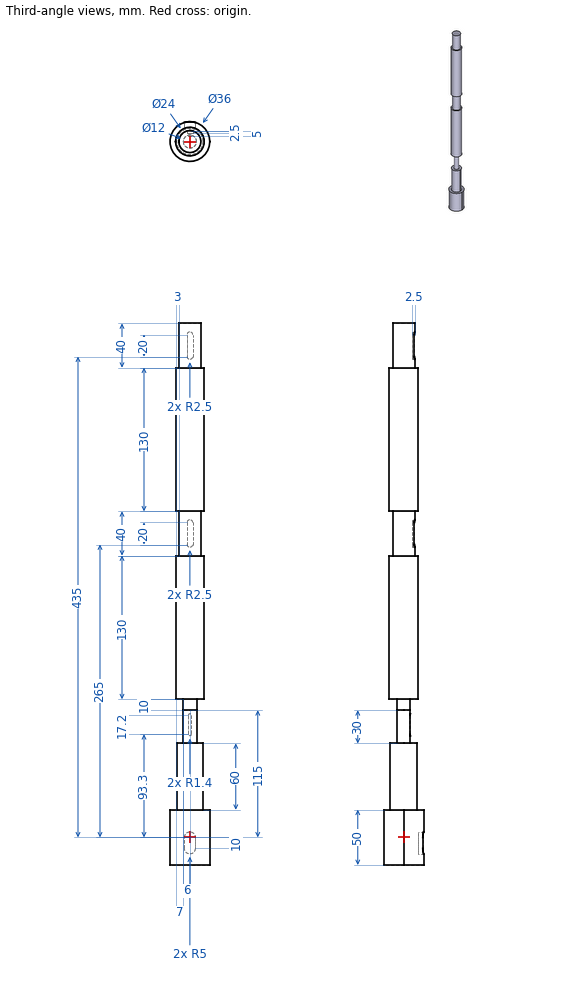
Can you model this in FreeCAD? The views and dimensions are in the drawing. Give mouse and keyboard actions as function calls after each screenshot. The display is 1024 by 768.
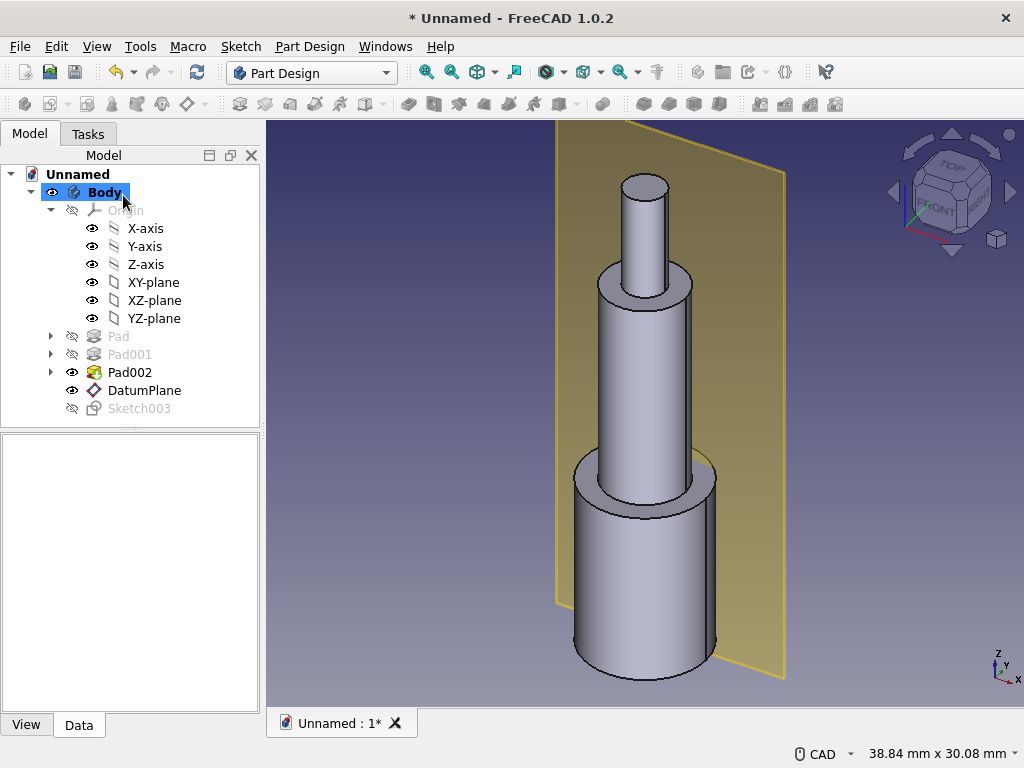
click(409, 104)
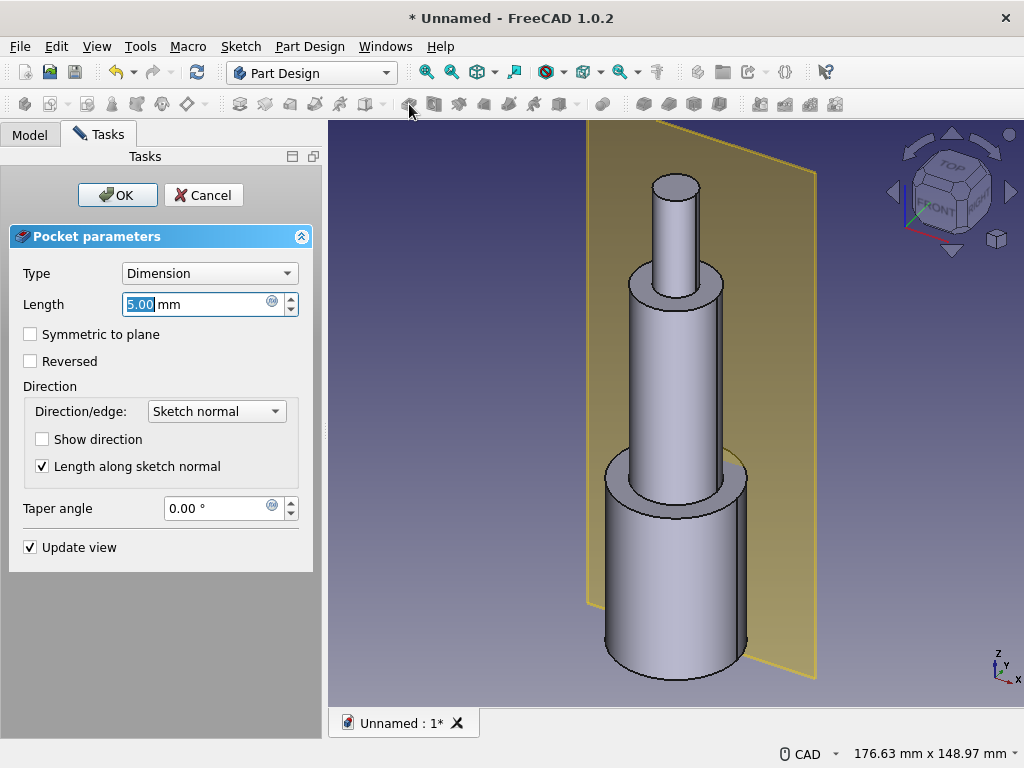
text(10)
key(Tab)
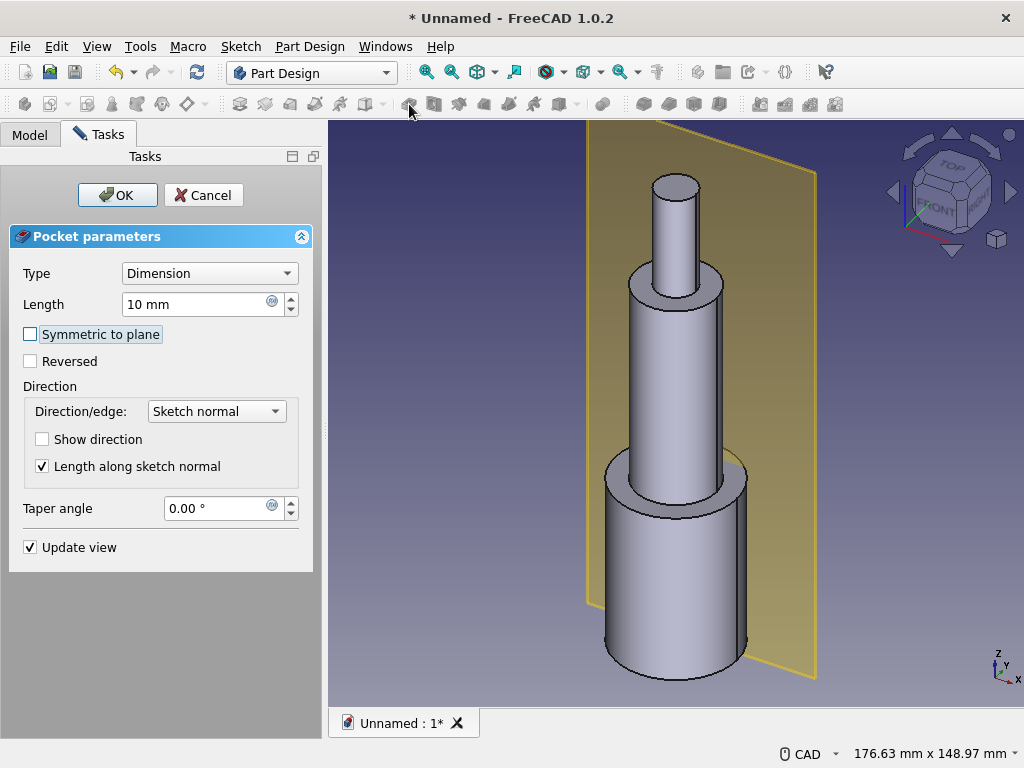
click(118, 195)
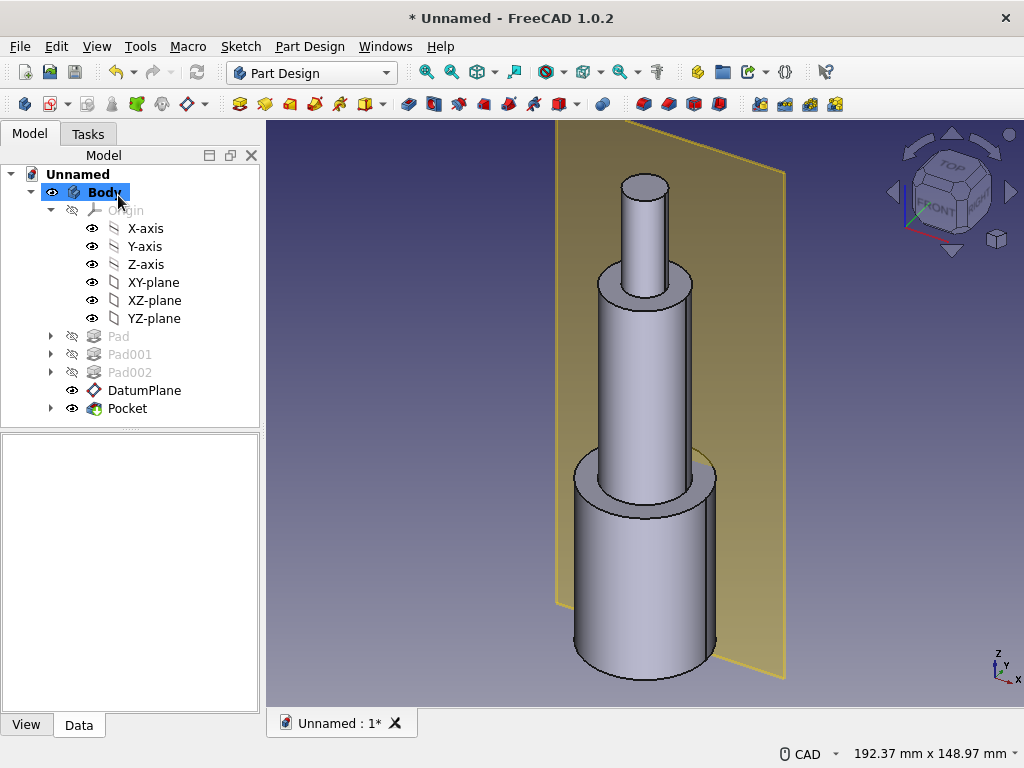
click(117, 390)
key(space)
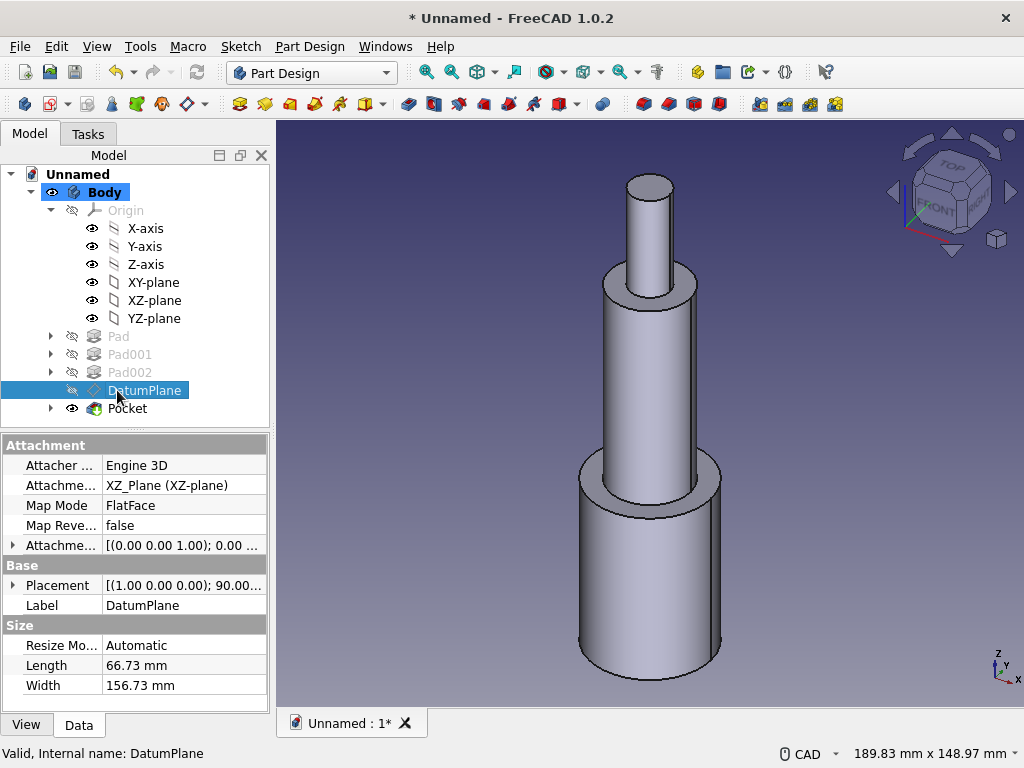
click(137, 300)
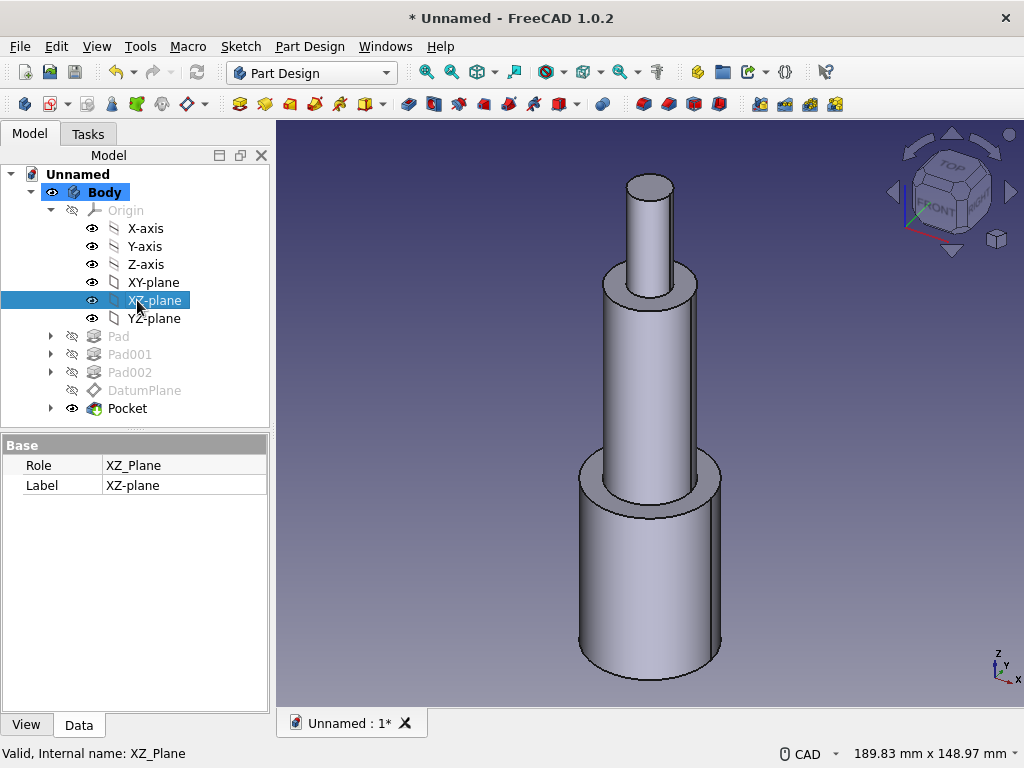
click(186, 104)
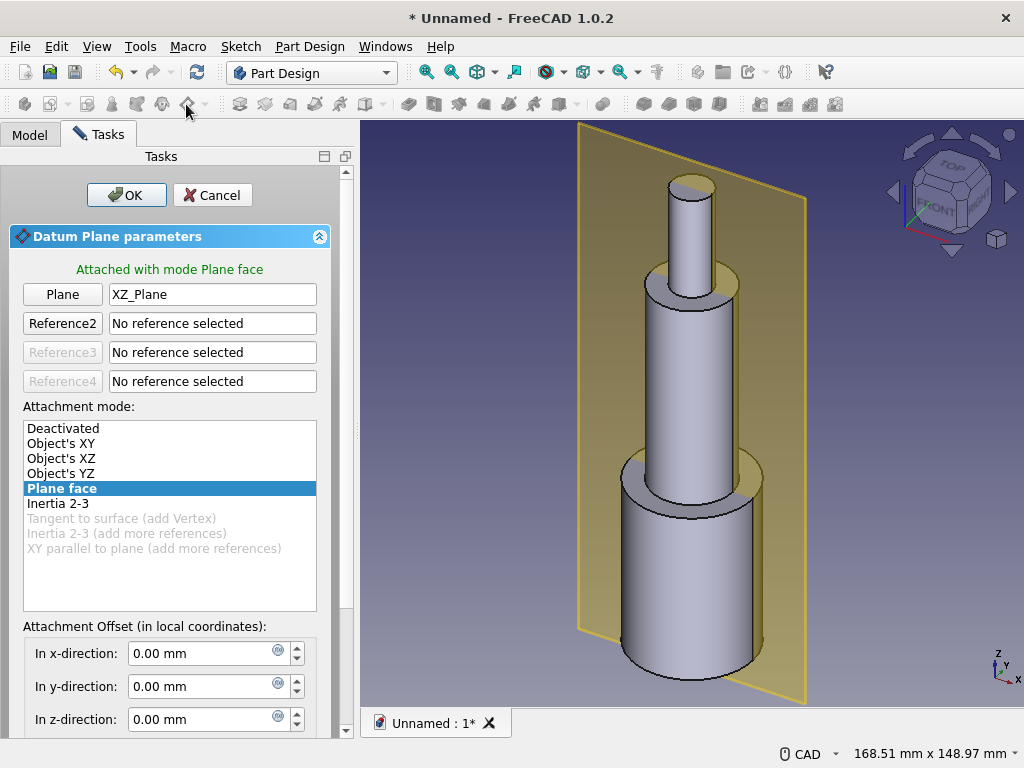
triple_click(210, 720)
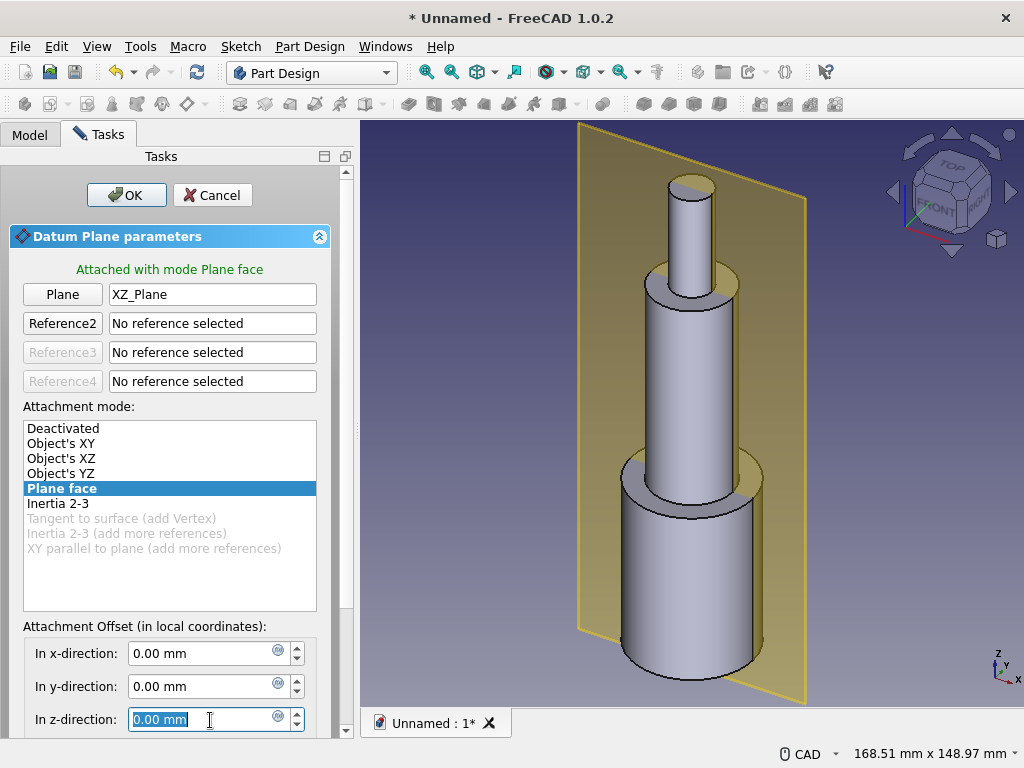
text(-5)
key(Tab)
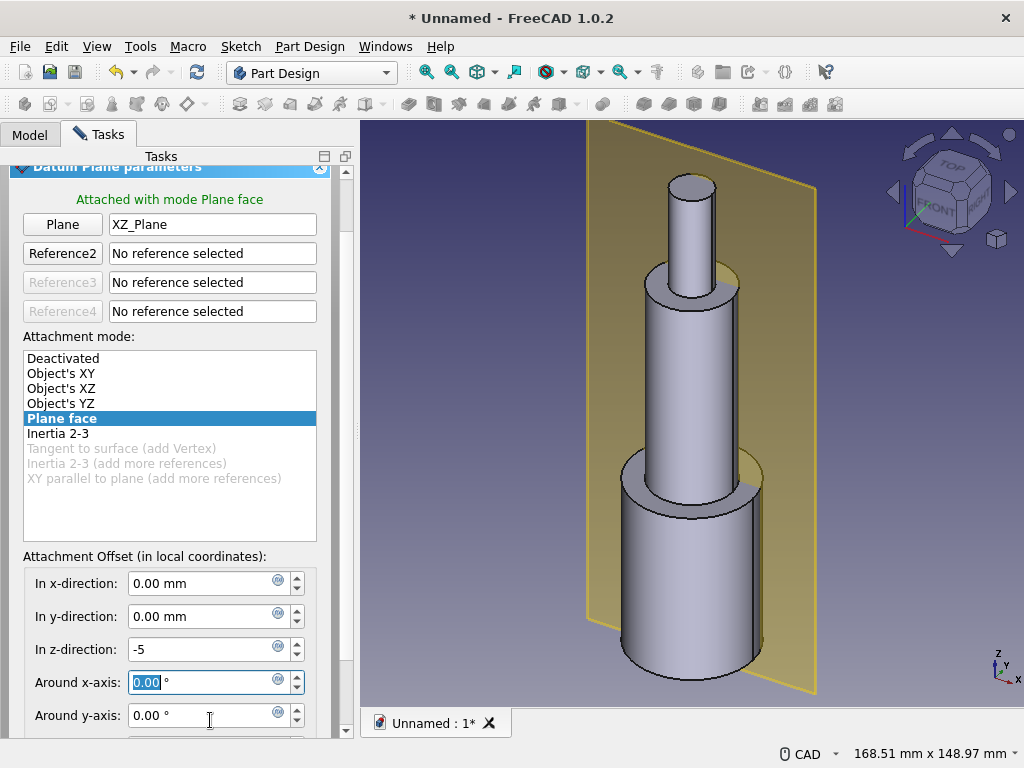
scroll(346, 452, up, 2)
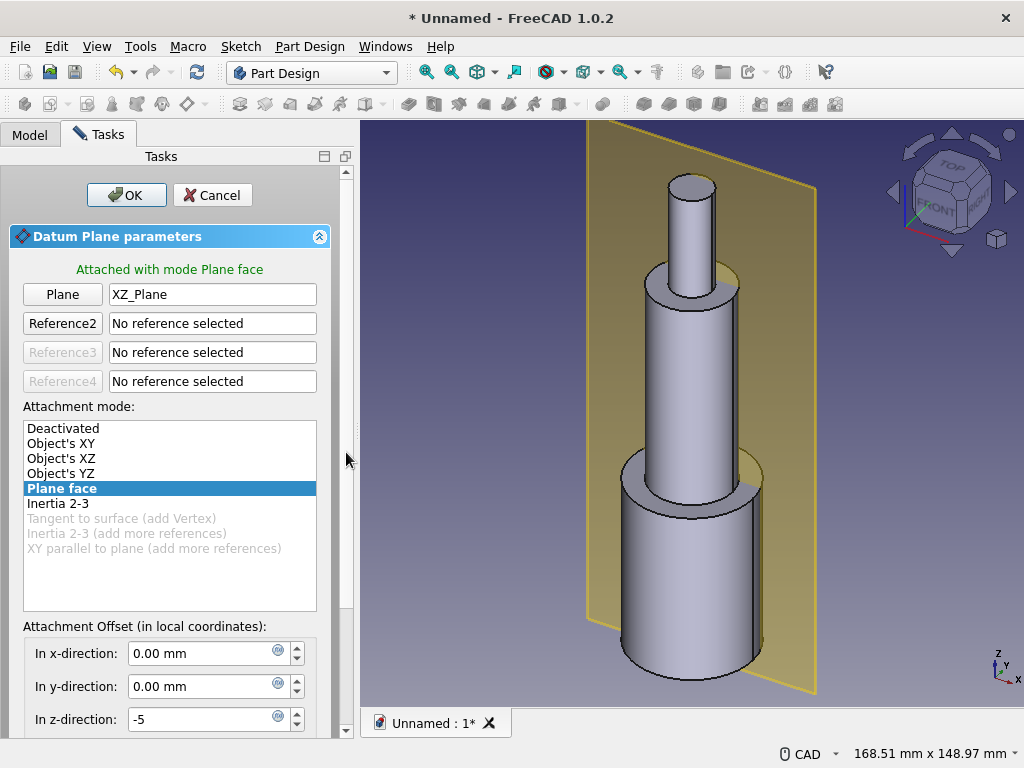
click(127, 195)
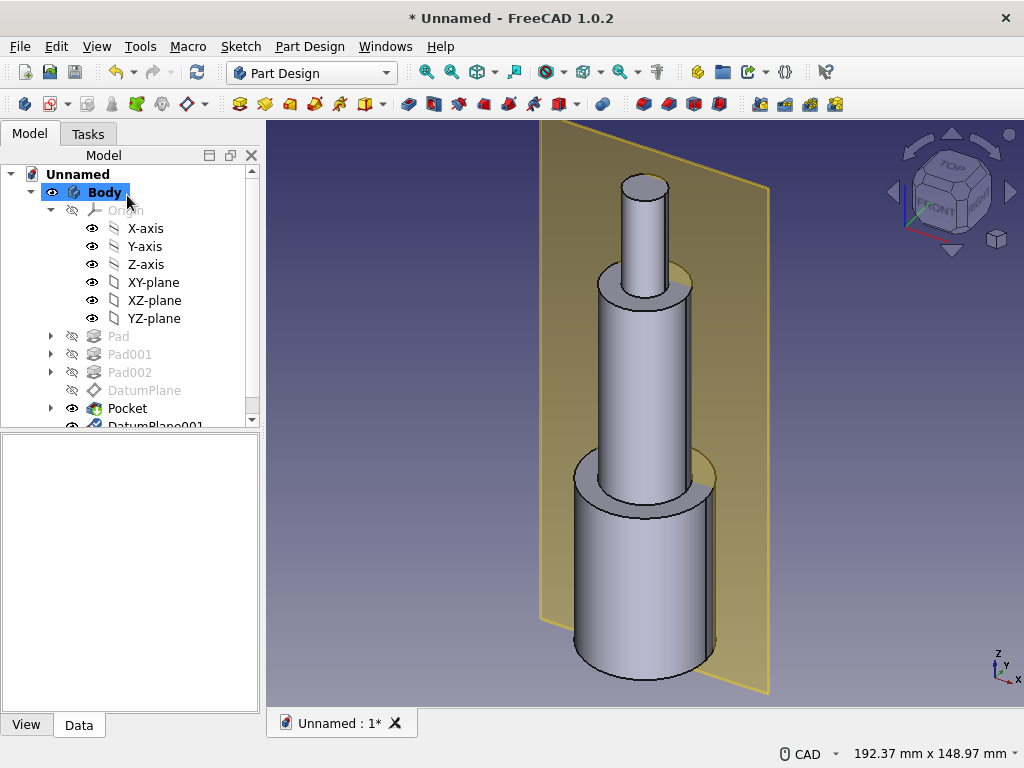
click(117, 426)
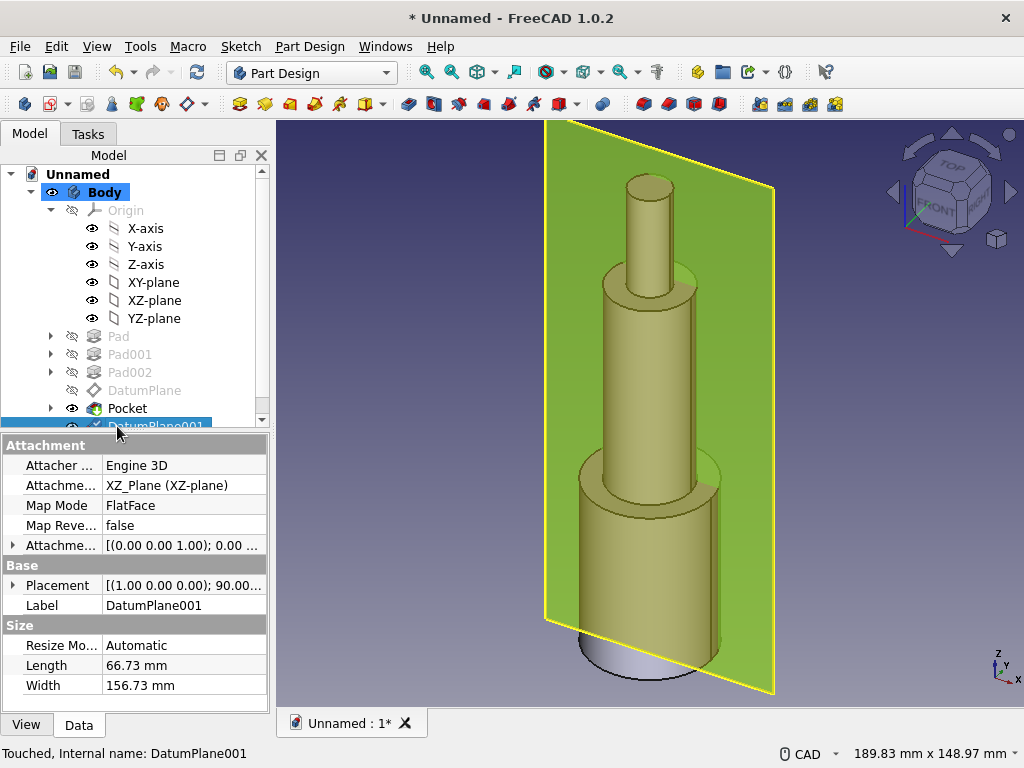
click(50, 104)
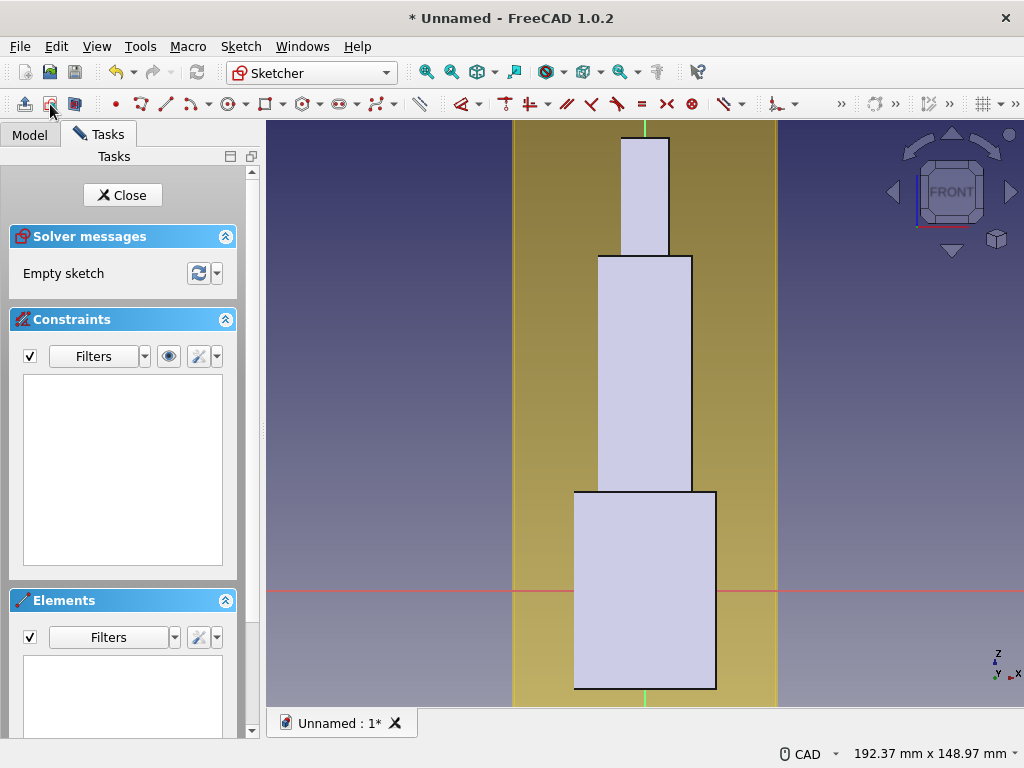
click(75, 104)